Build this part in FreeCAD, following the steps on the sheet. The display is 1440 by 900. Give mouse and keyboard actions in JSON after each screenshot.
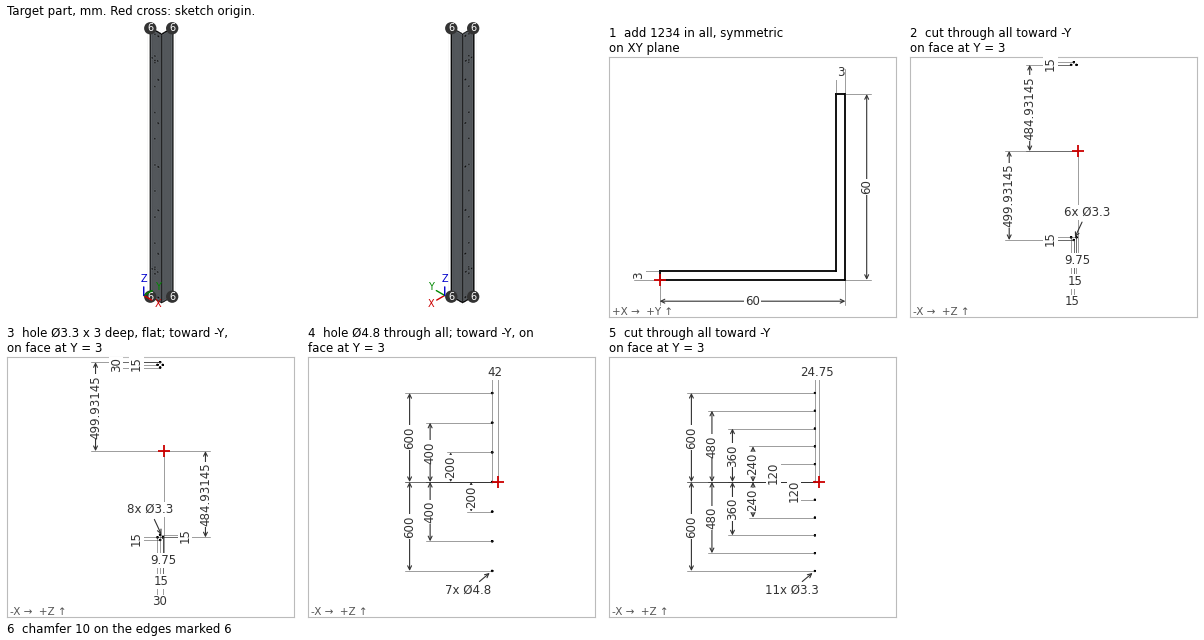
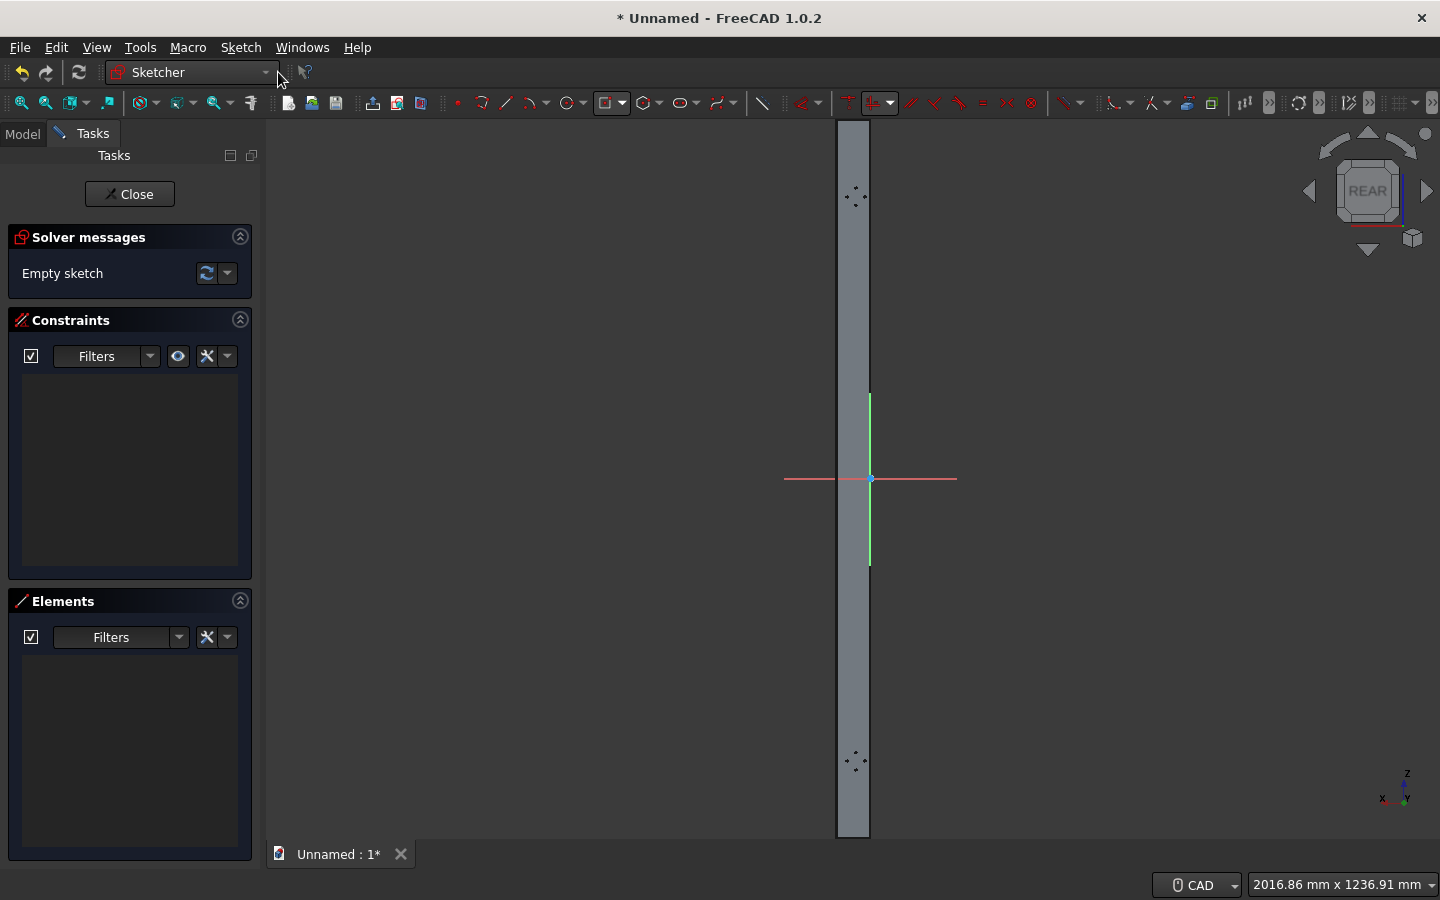
{"action": "left_click", "coordinate": [422, 104]}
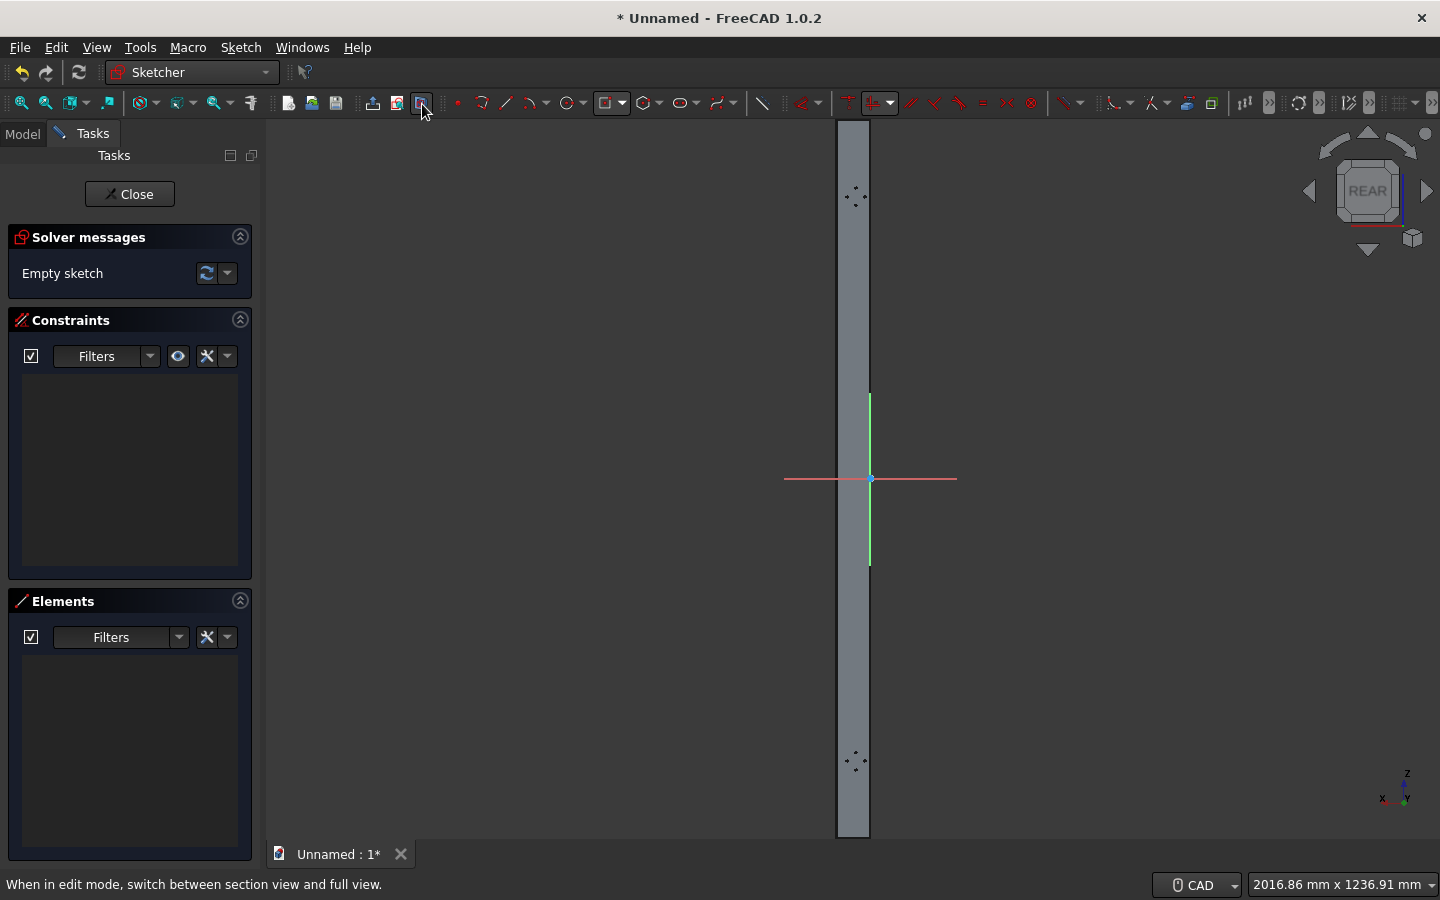
{"action": "scroll", "coordinate": [636, 479], "scroll_direction": "down", "scroll_amount": 2}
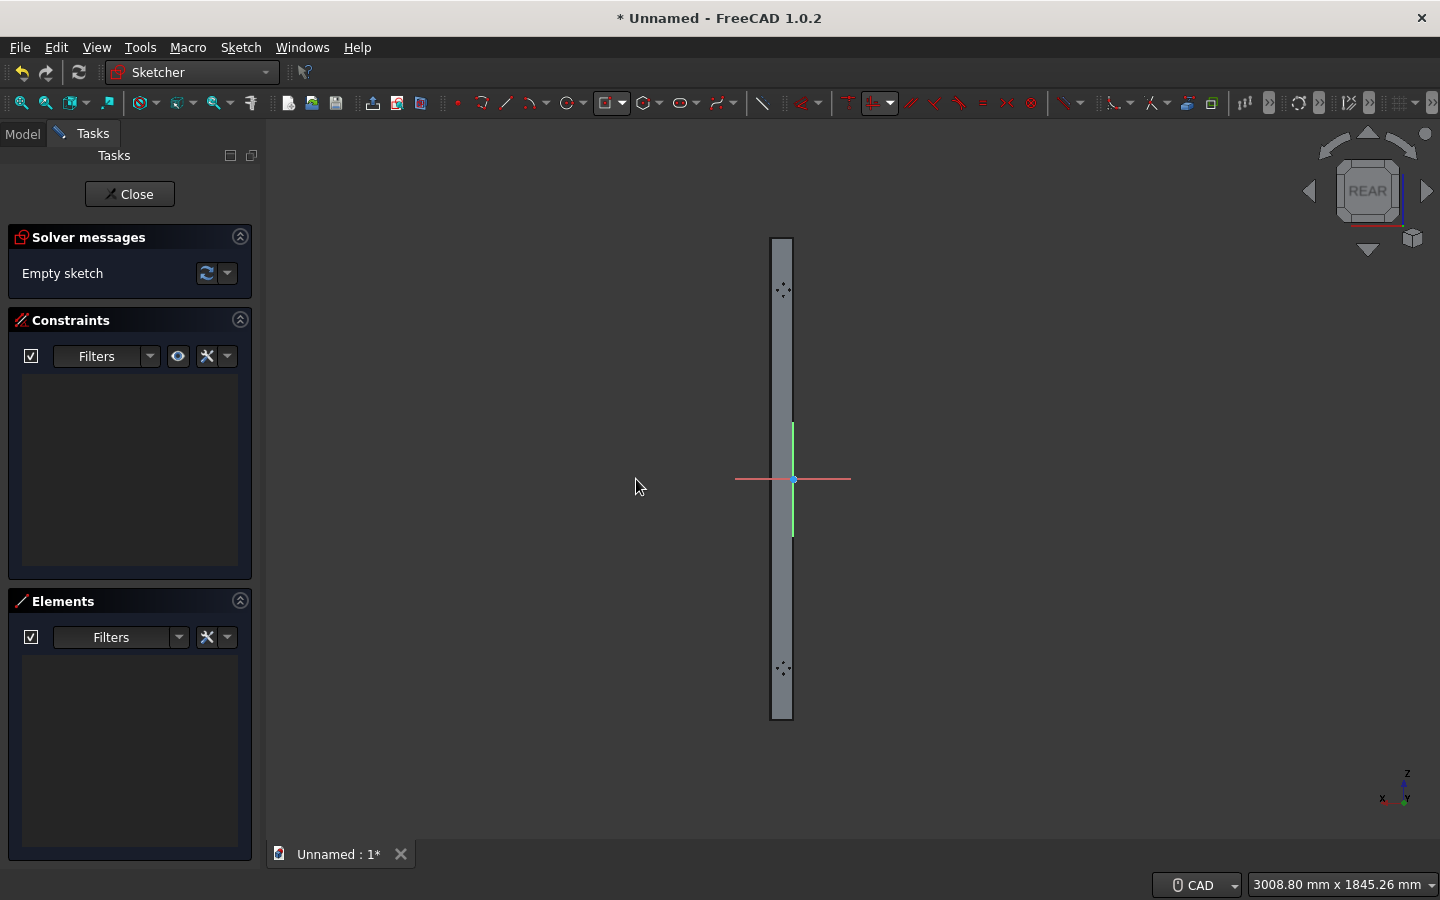
{"action": "left_click", "coordinate": [568, 104]}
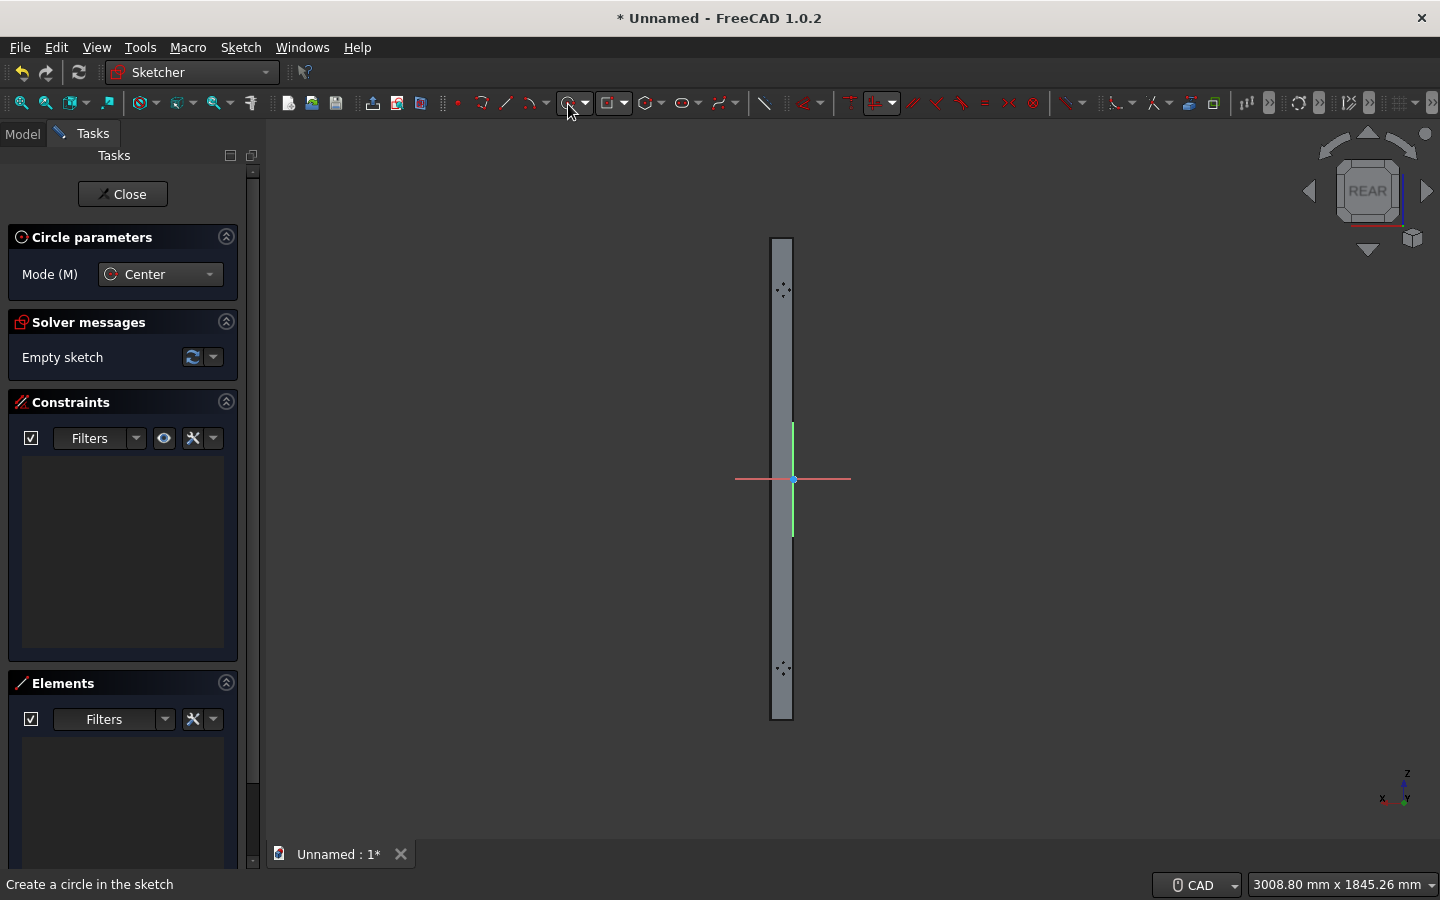
{"action": "scroll", "coordinate": [777, 479], "scroll_direction": "up", "scroll_amount": 16}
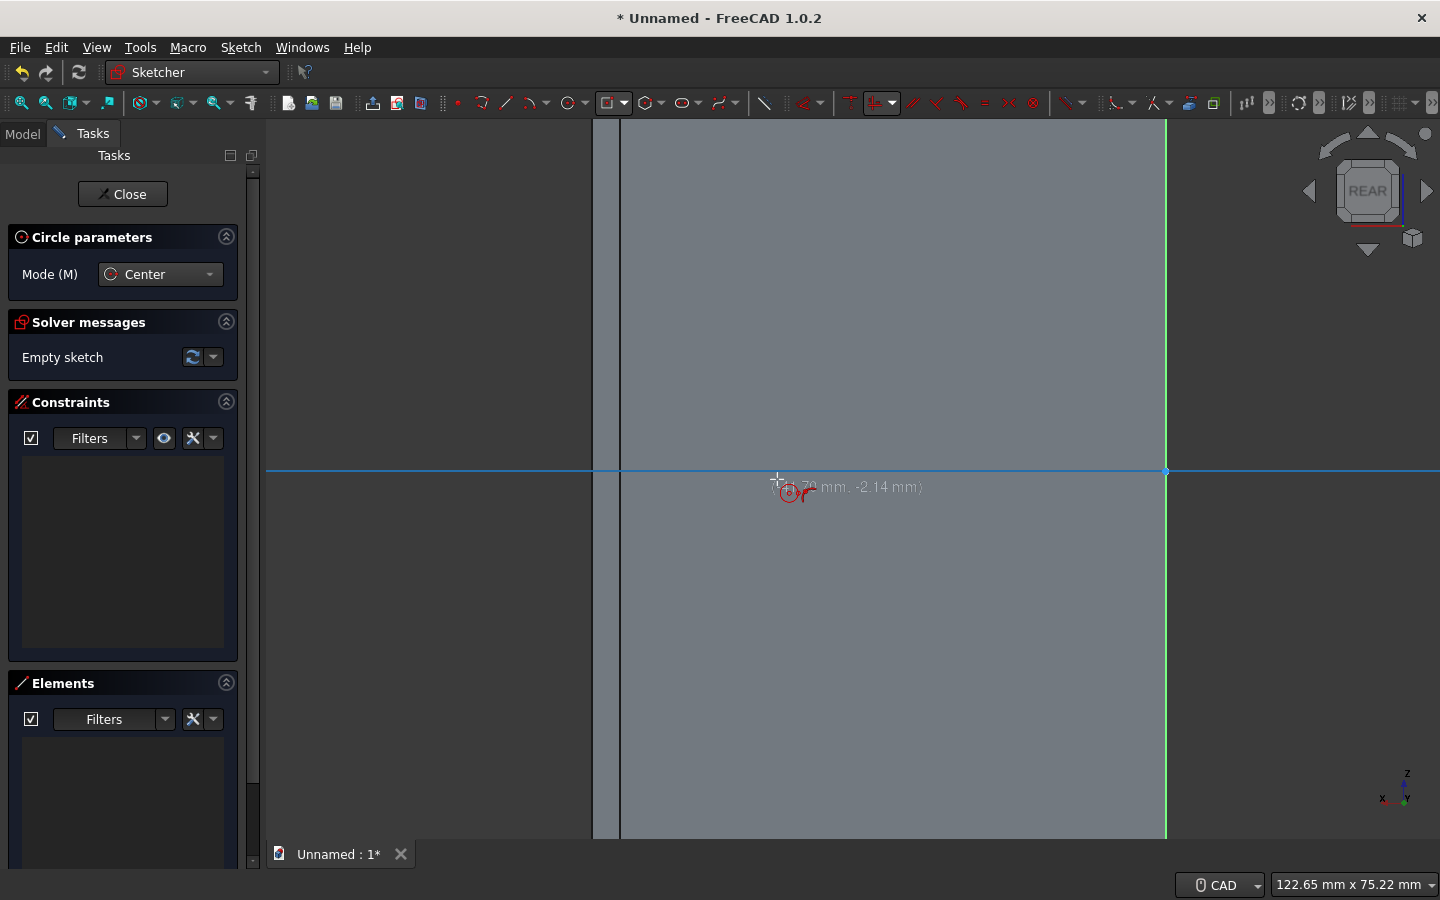
{"action": "scroll", "coordinate": [776, 479], "scroll_direction": "down", "scroll_amount": 15}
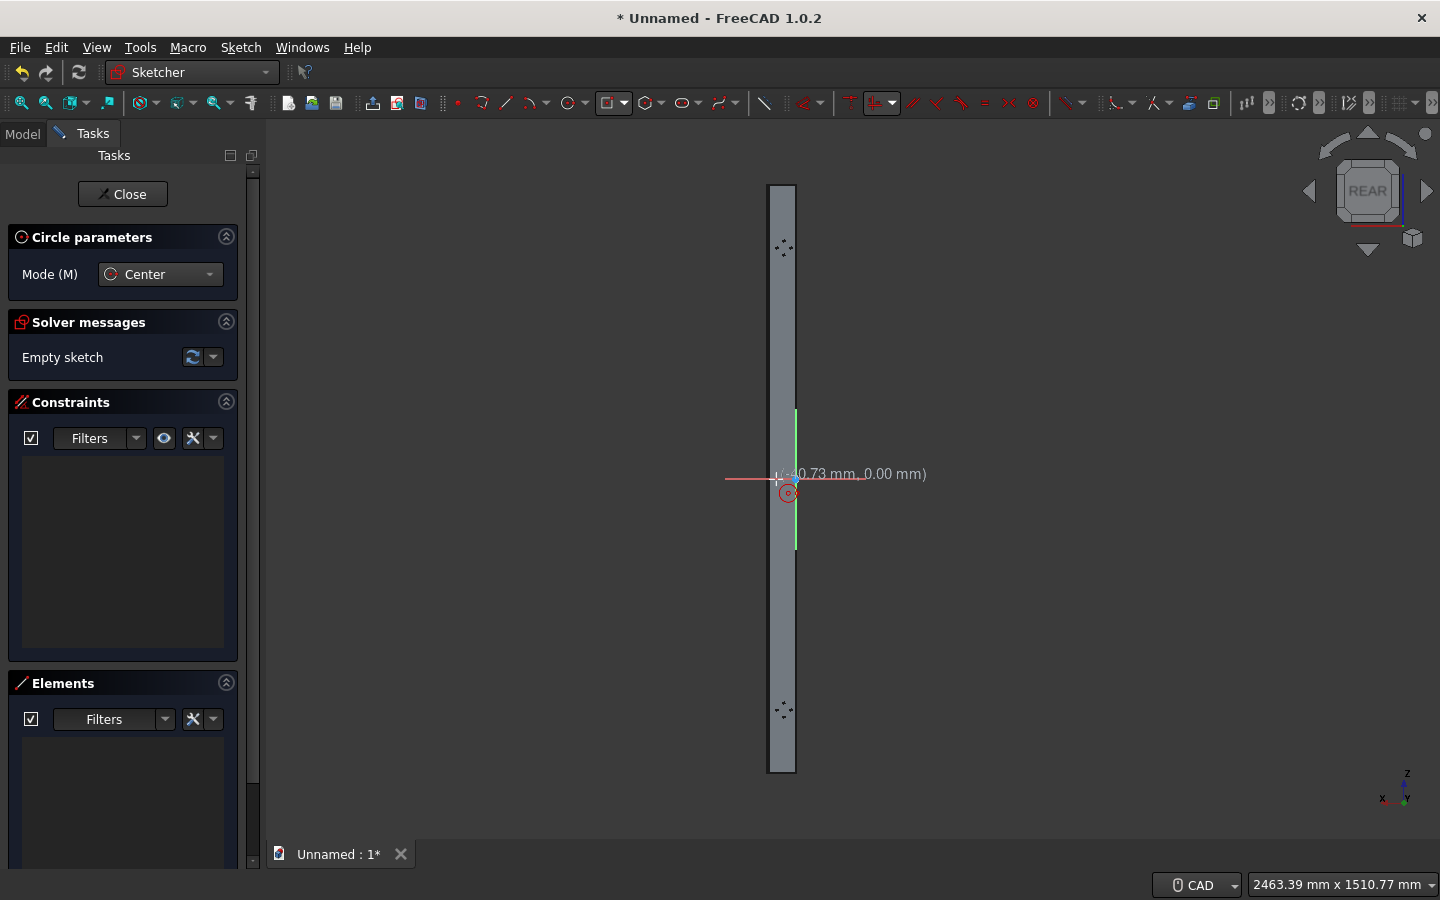
{"action": "left_click", "coordinate": [776, 479]}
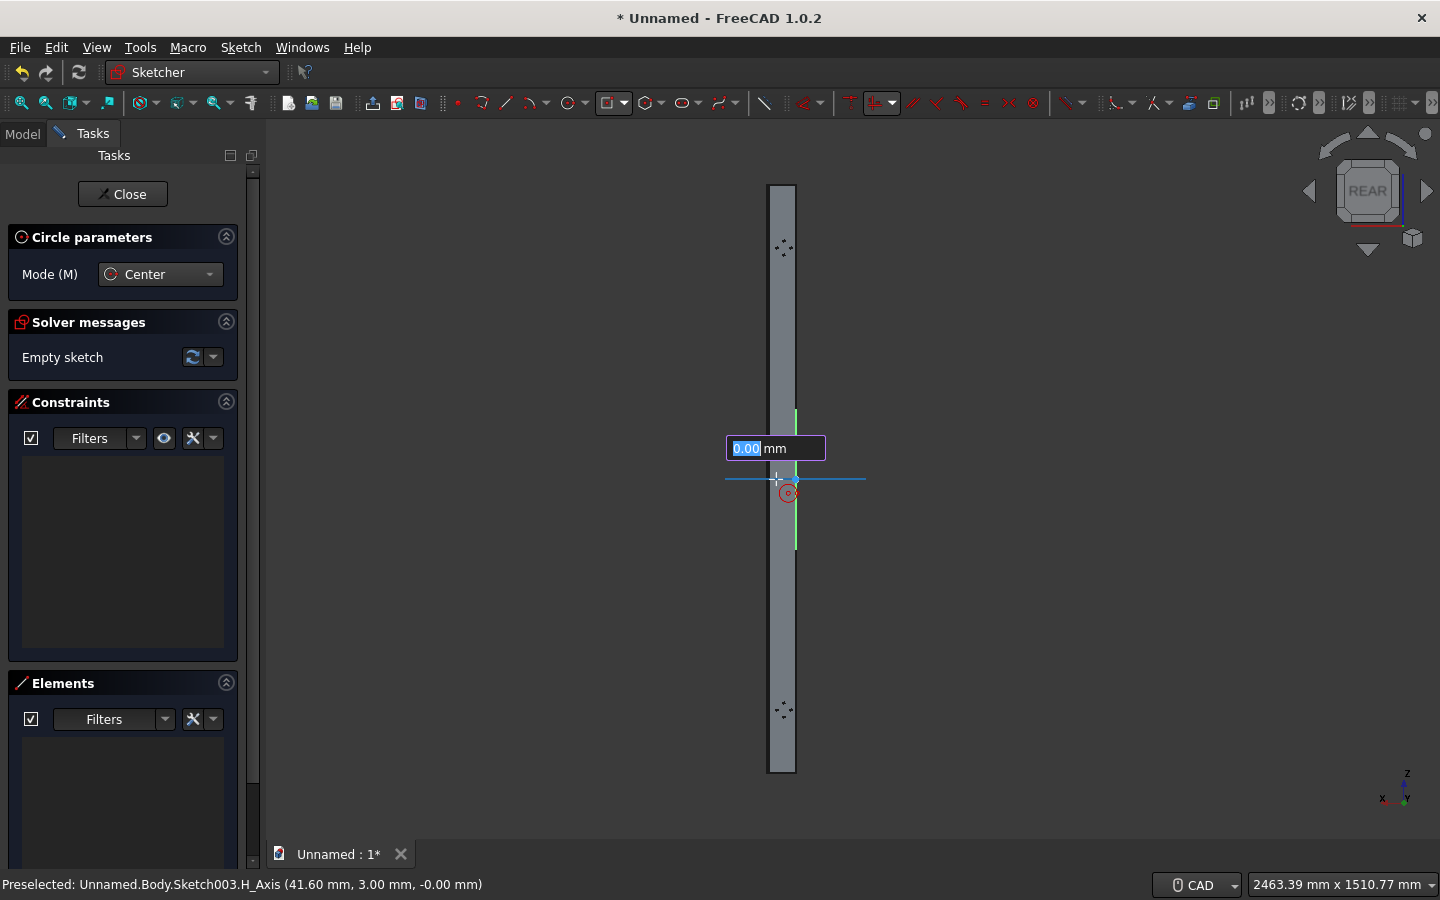
{"action": "scroll", "coordinate": [776, 478], "scroll_direction": "up", "scroll_amount": 14}
{"action": "mouse_move", "coordinate": [773, 471]}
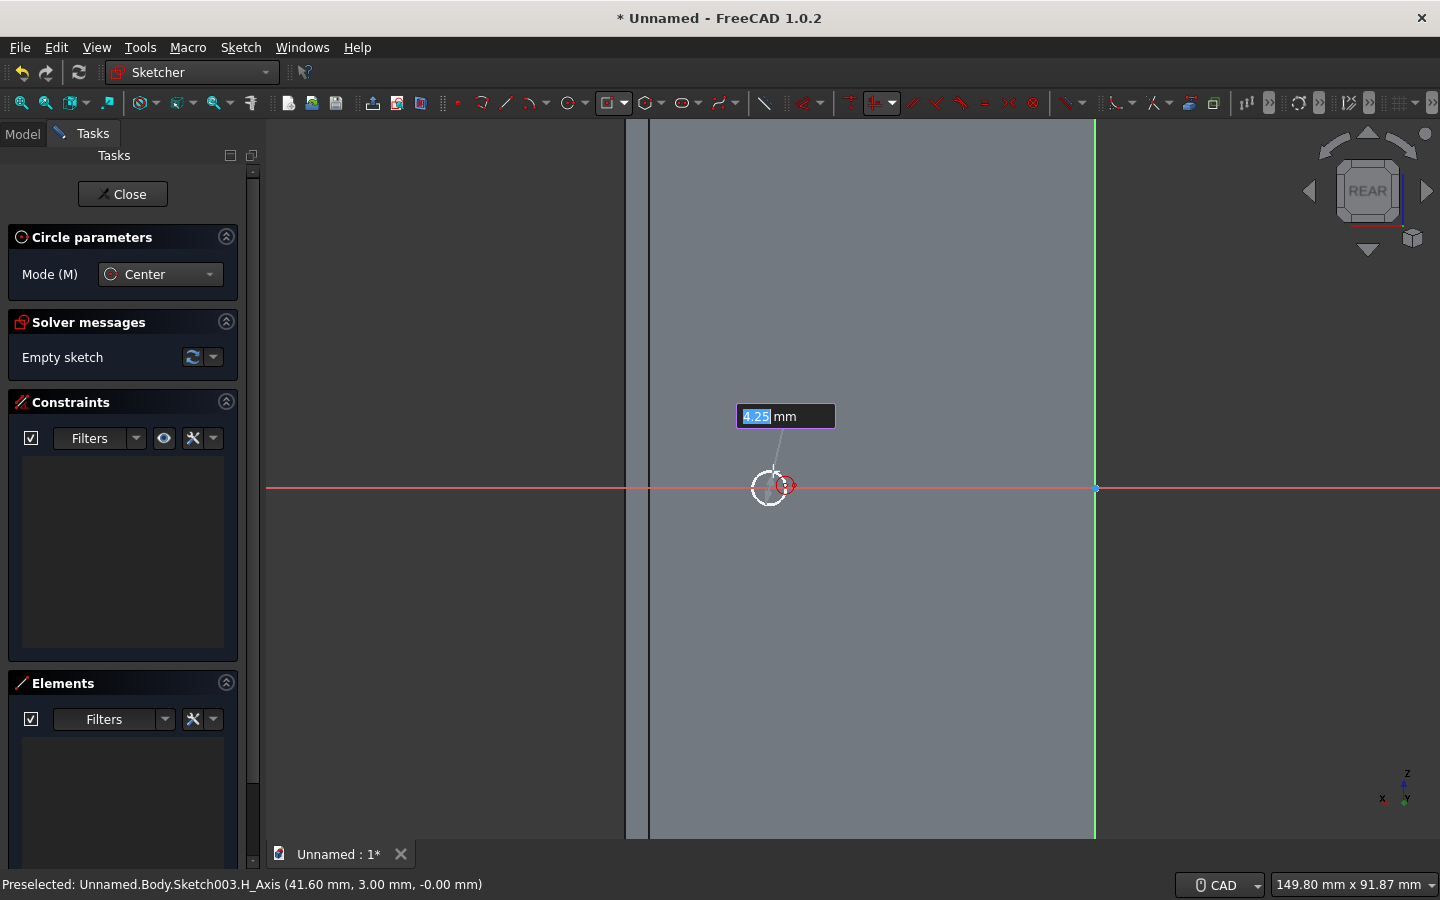
{"action": "type", "text": "4.8"}
{"action": "key", "text": "Return"}